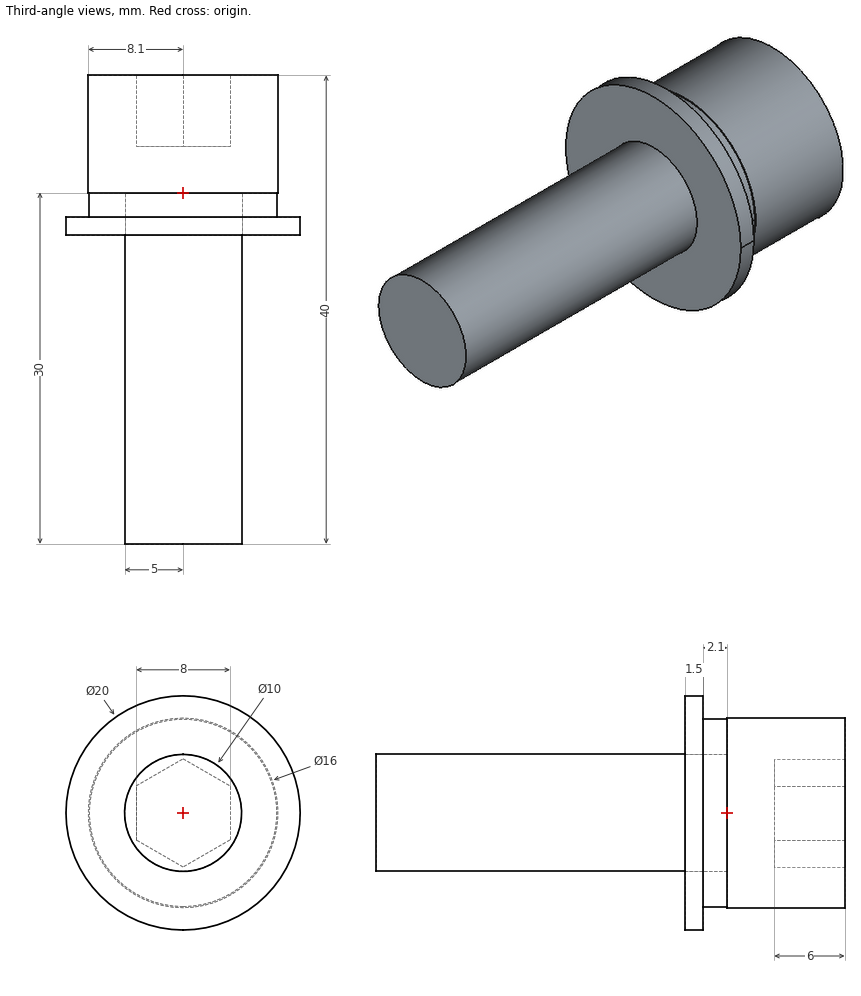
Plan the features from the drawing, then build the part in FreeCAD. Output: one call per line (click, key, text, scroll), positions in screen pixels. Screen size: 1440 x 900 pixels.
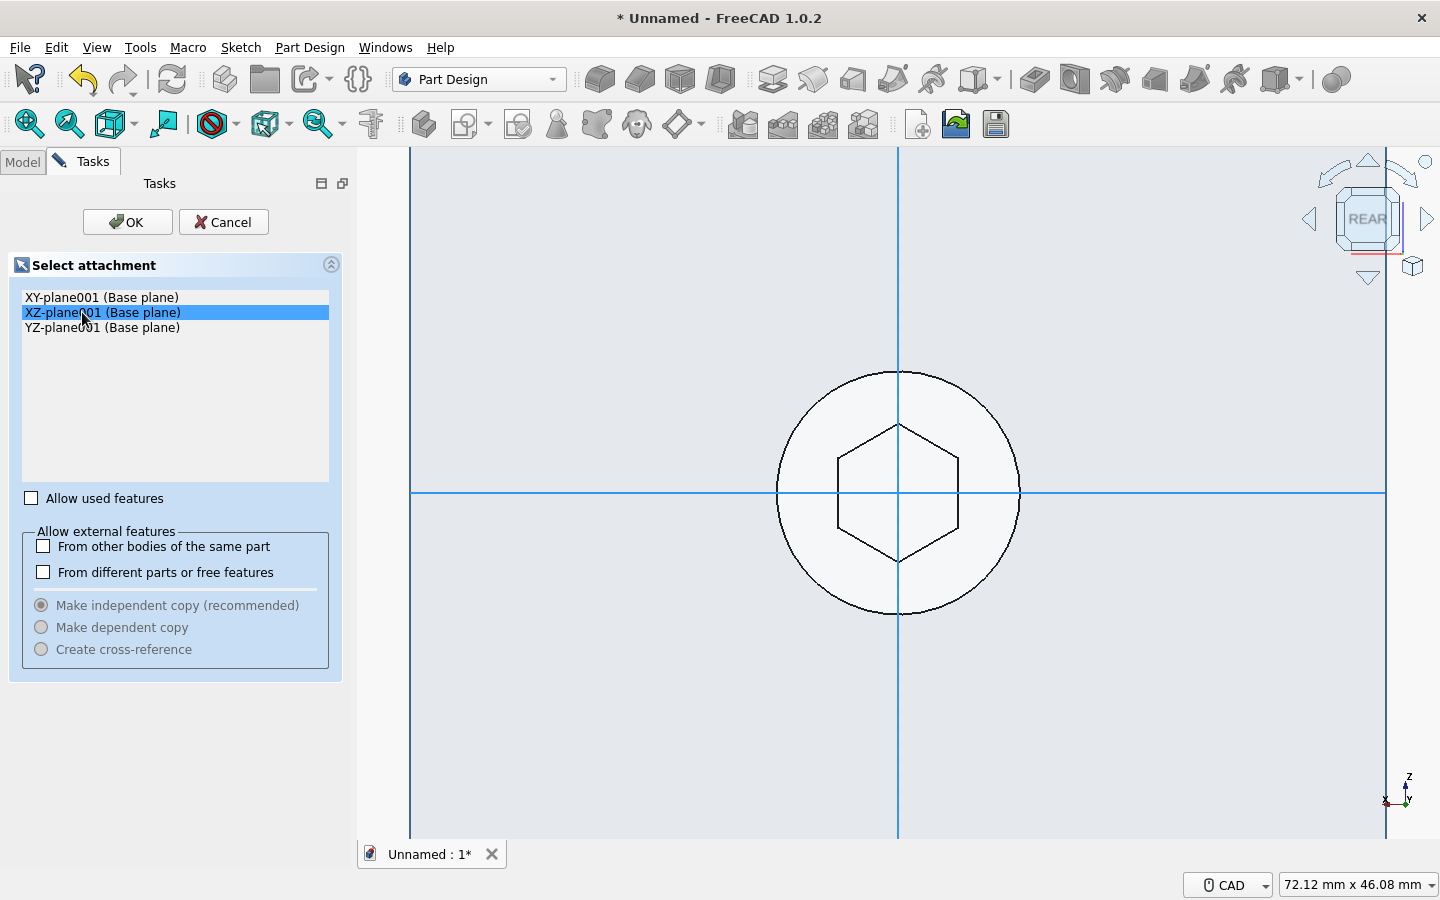
click(128, 222)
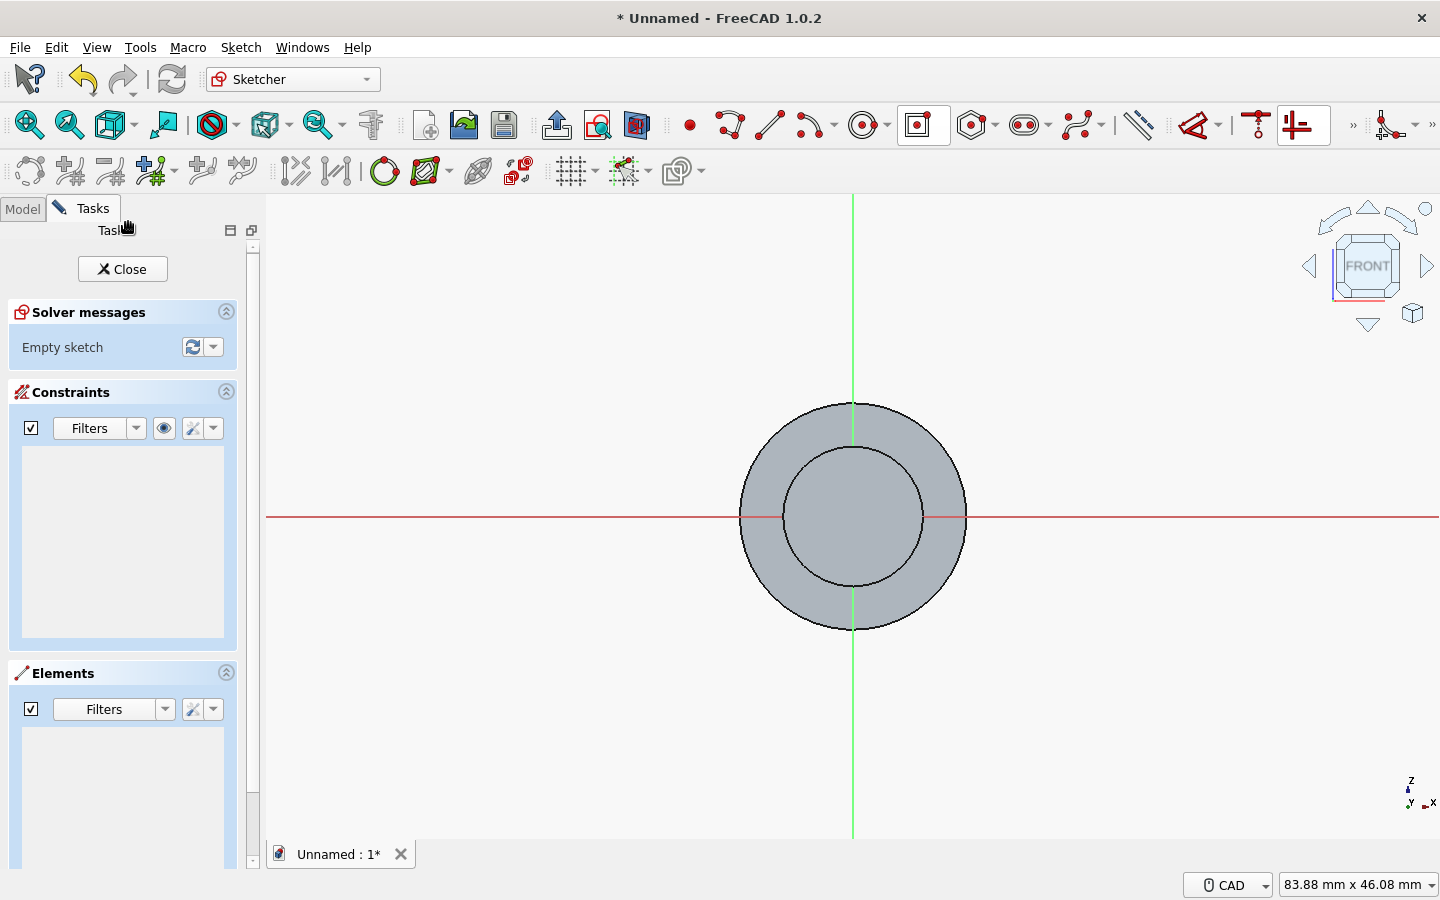
scroll(937, 516, up, 3)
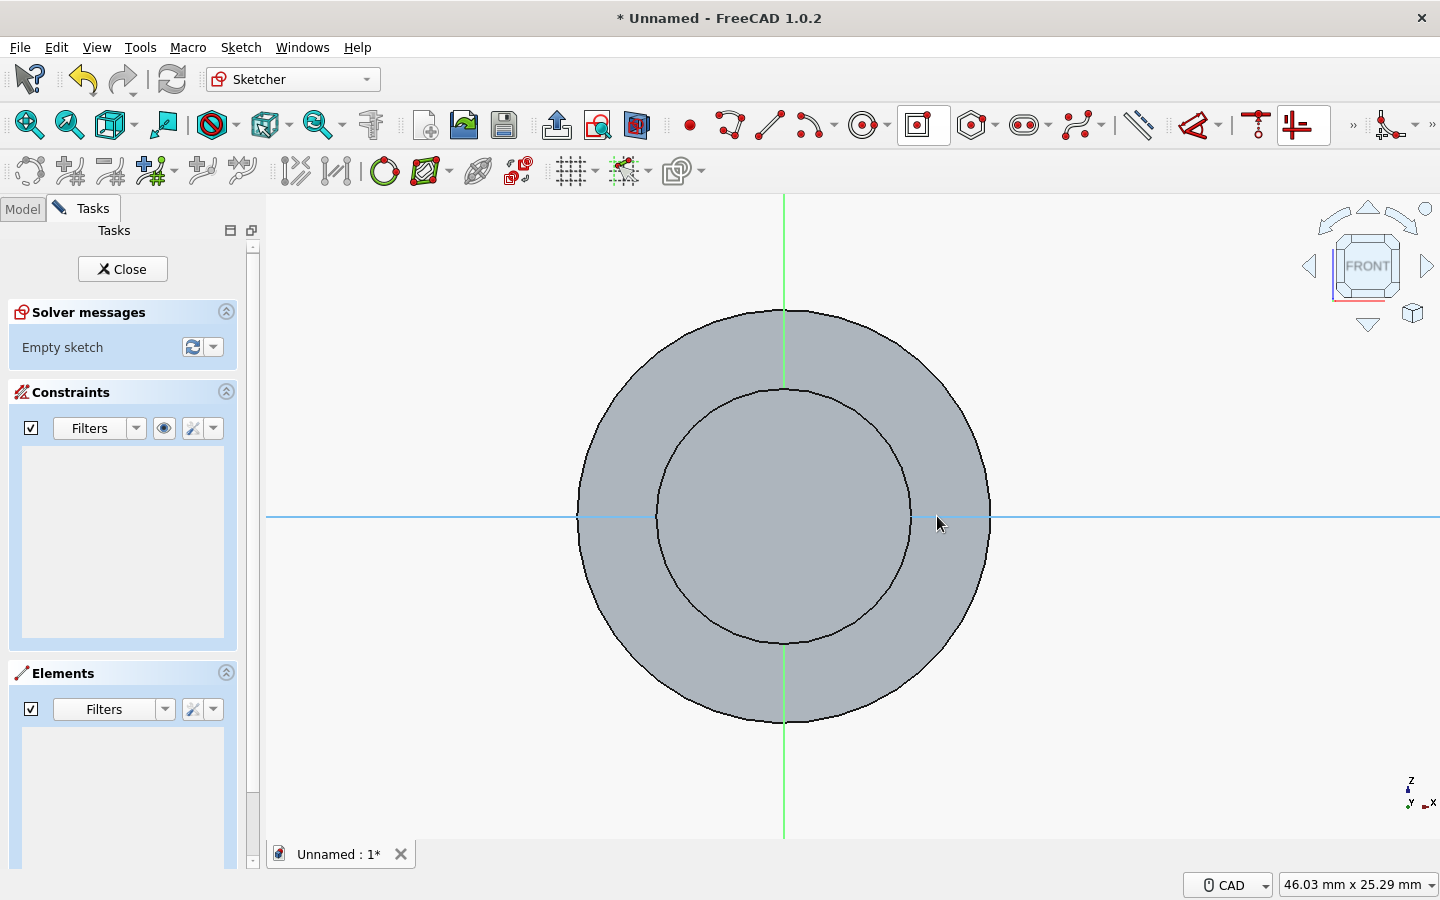
click(864, 126)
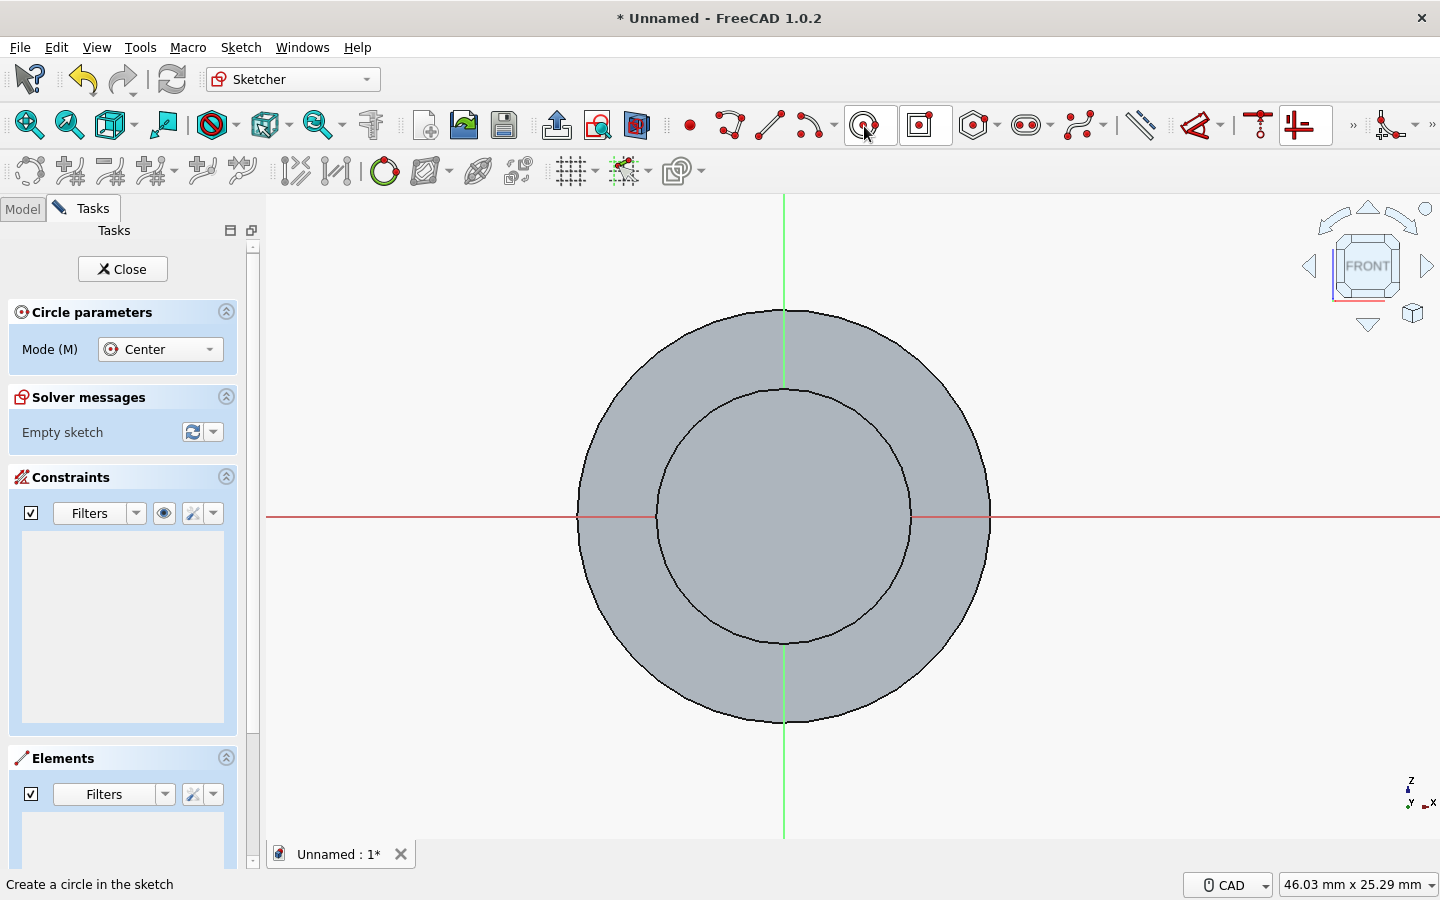
click(784, 516)
move(928, 372)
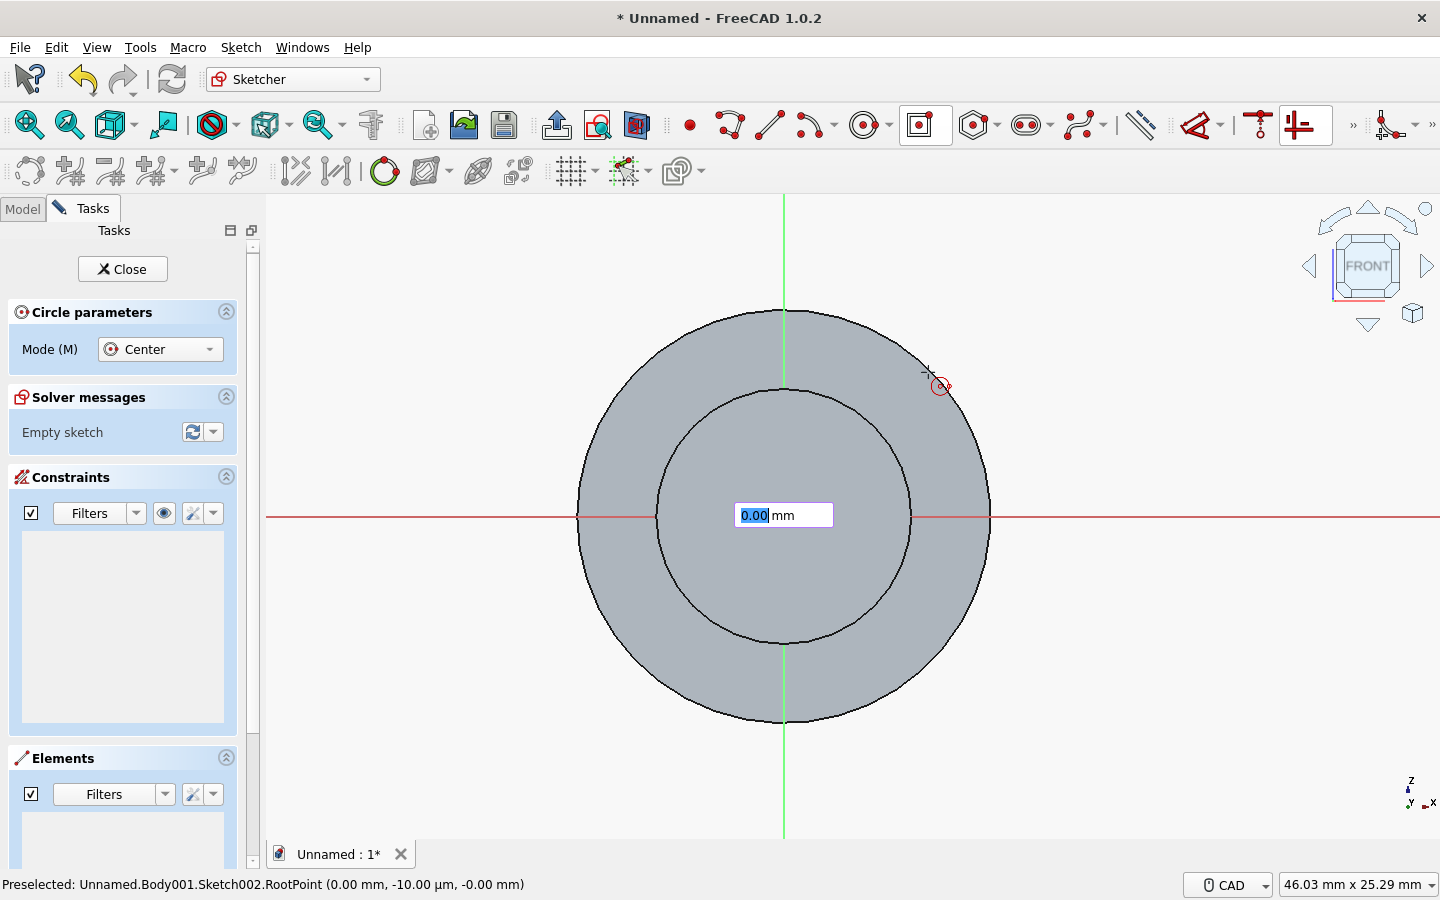
text(16)
key(Return)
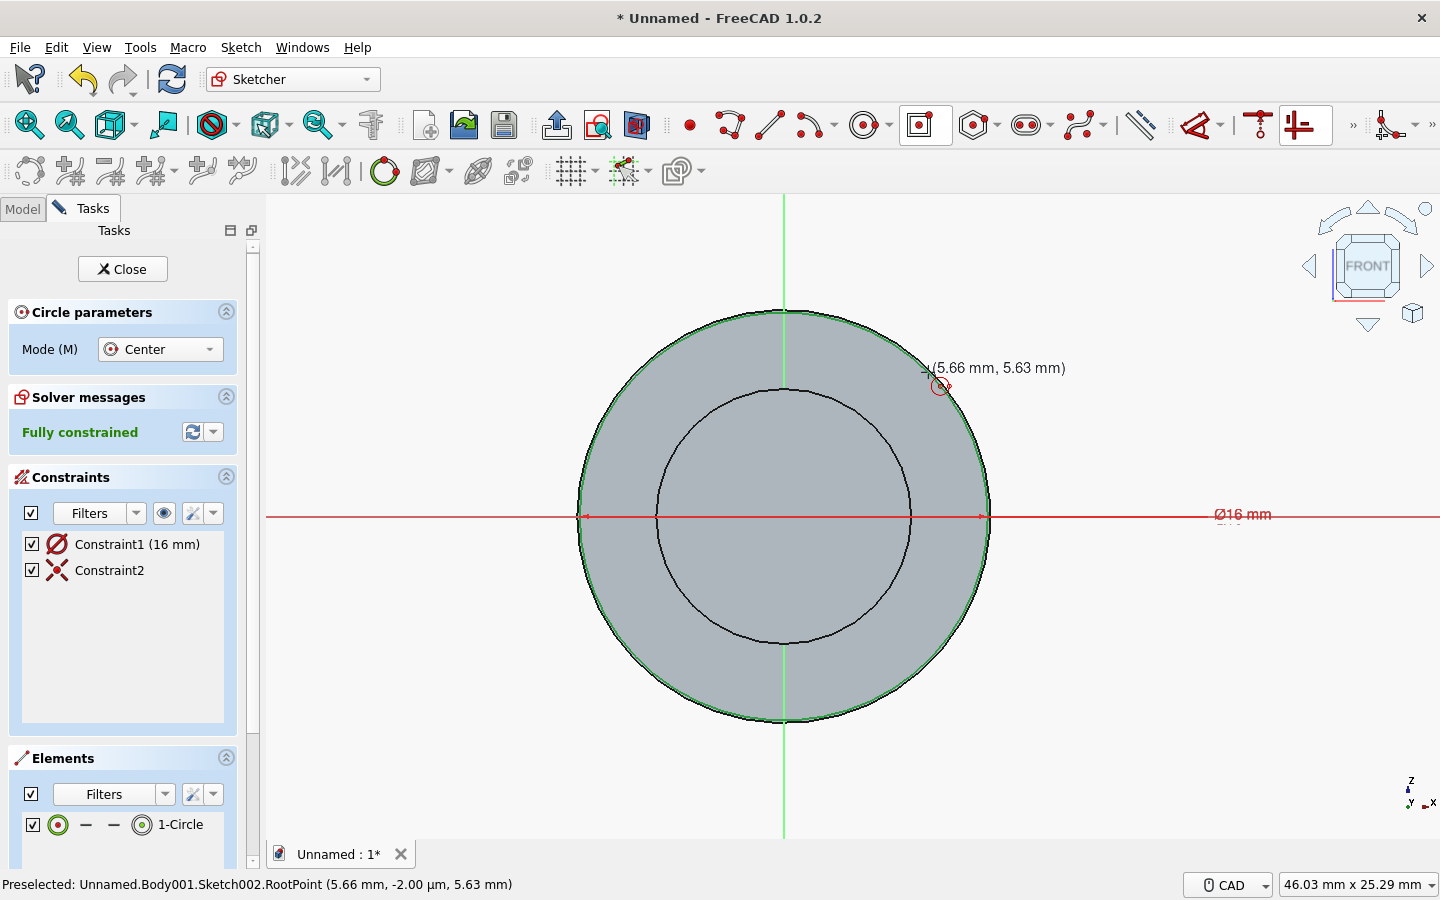
click(784, 516)
move(874, 426)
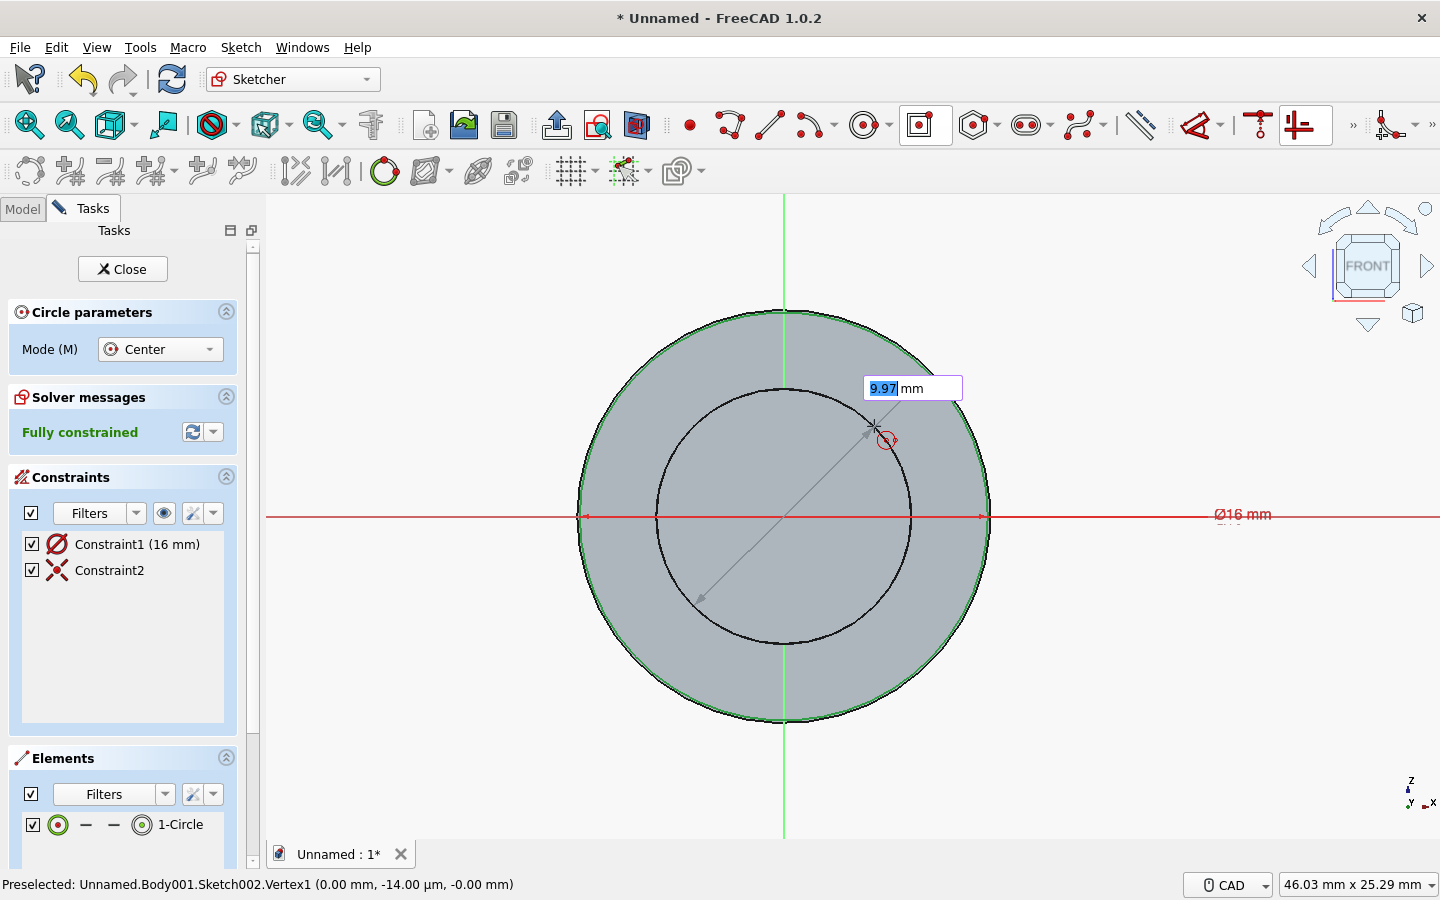
text(10)
key(Return)
key(Escape)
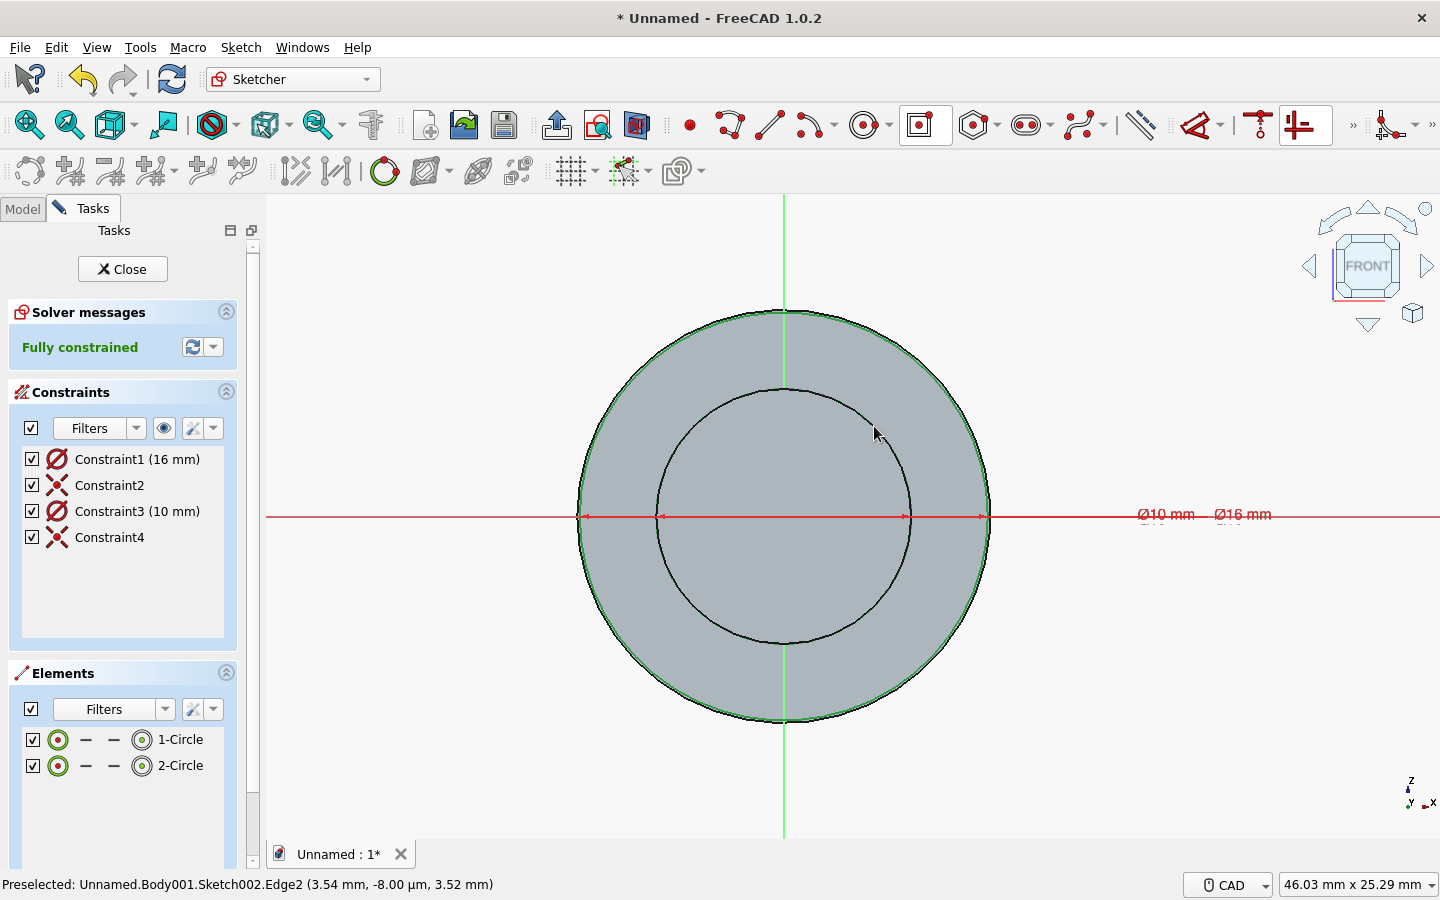
click(123, 269)